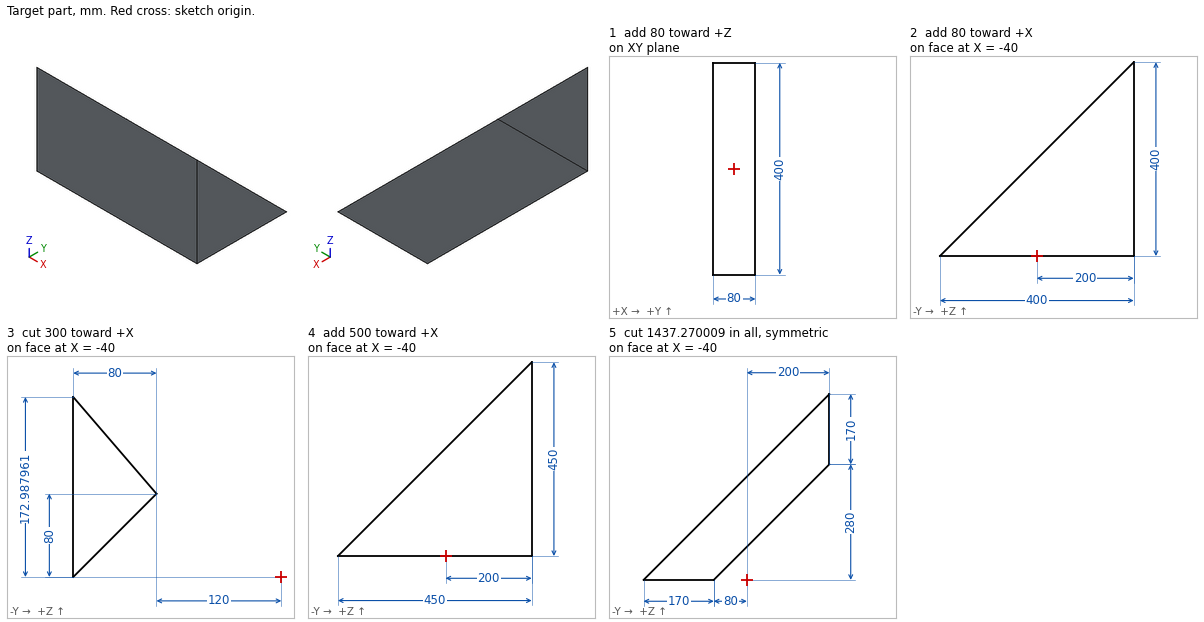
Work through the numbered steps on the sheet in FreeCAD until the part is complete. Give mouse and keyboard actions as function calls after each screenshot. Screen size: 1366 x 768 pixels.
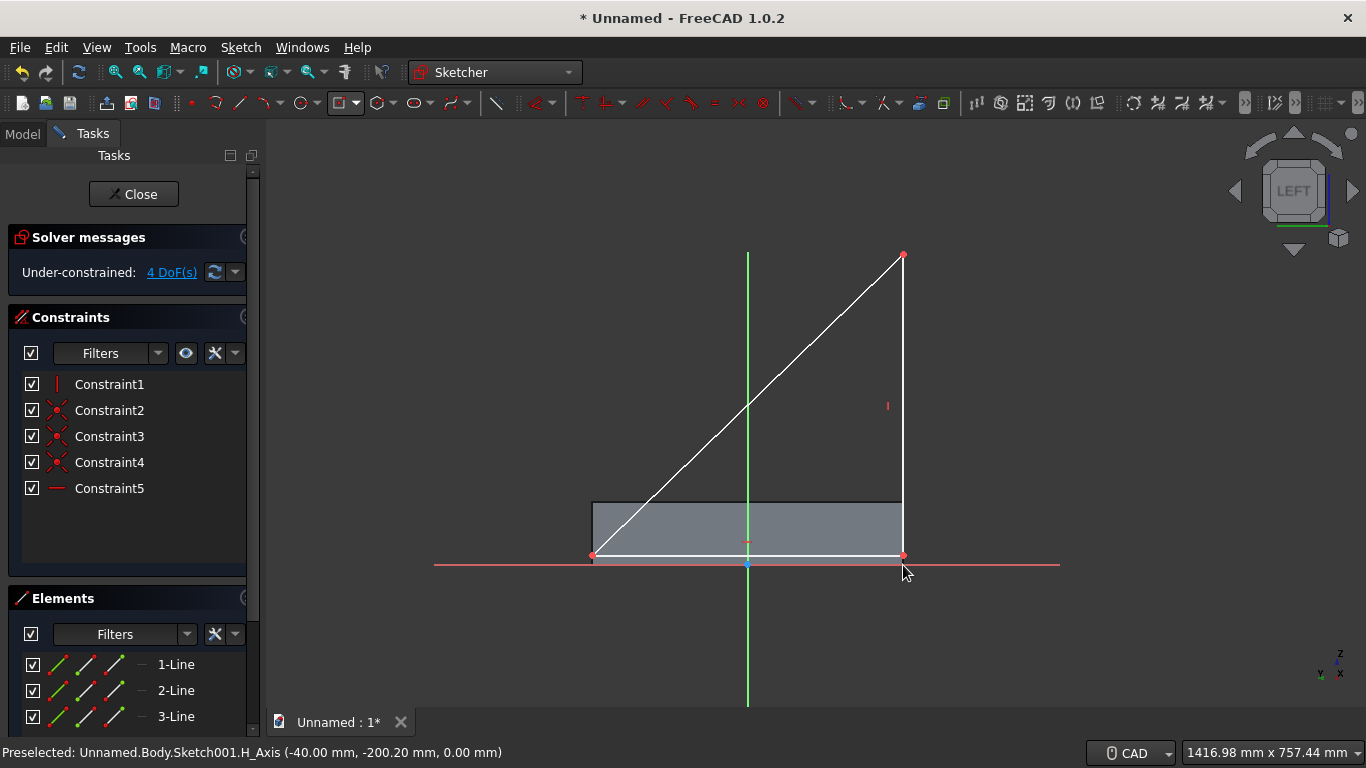
click(903, 556)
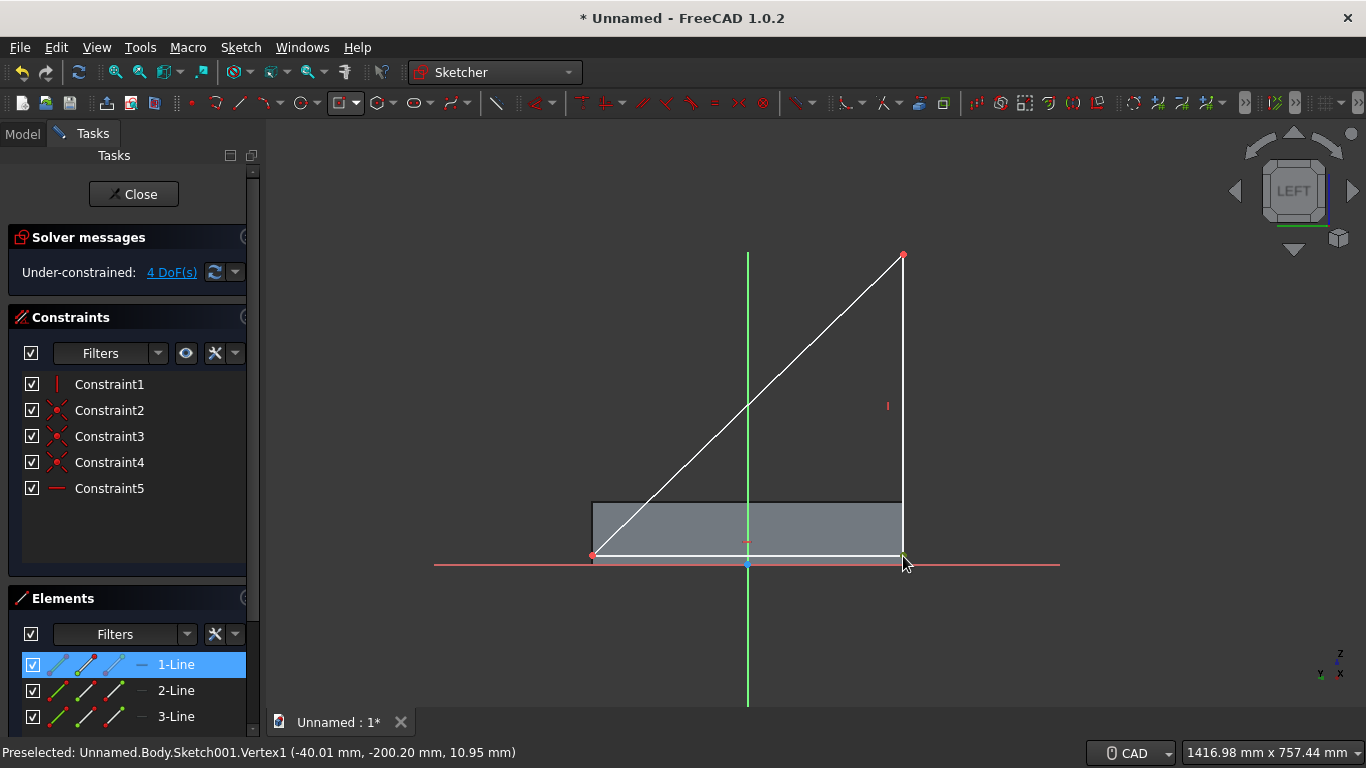
click(488, 564)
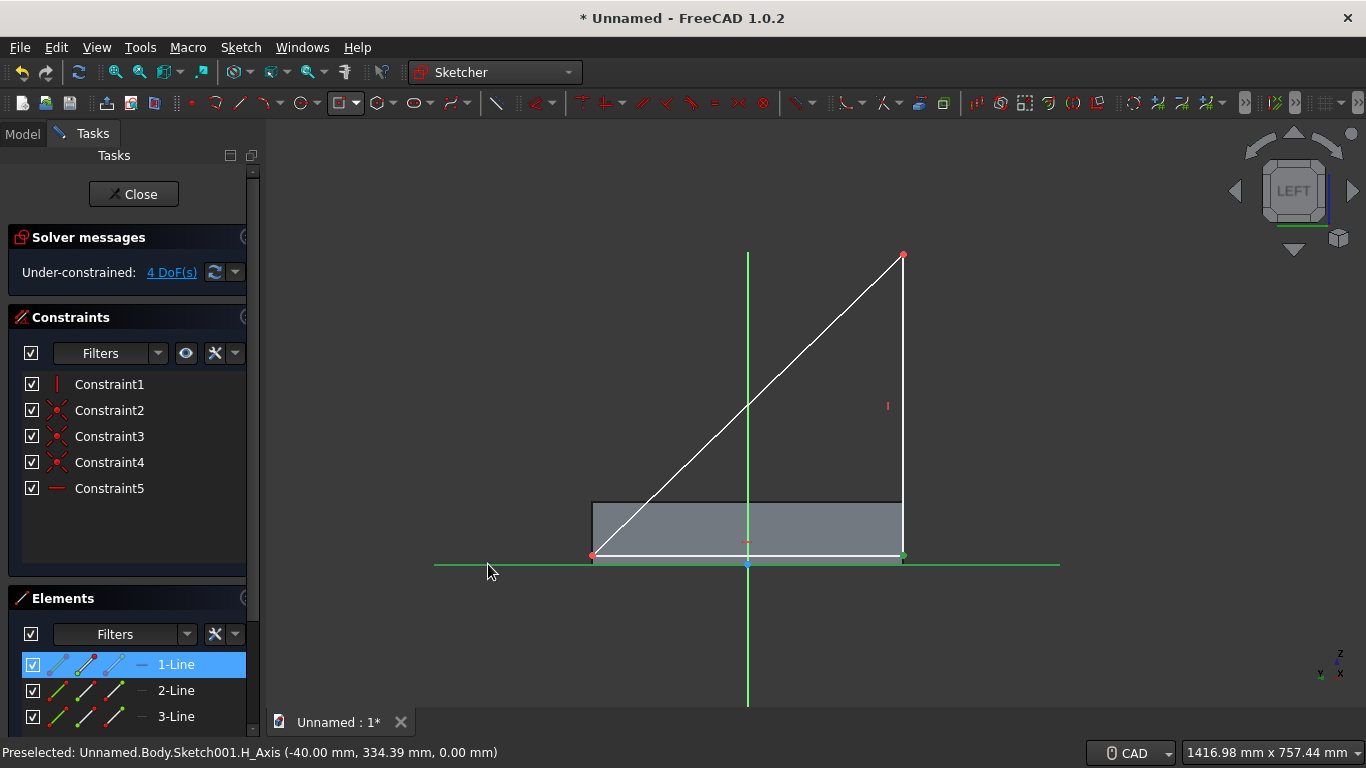
click(582, 104)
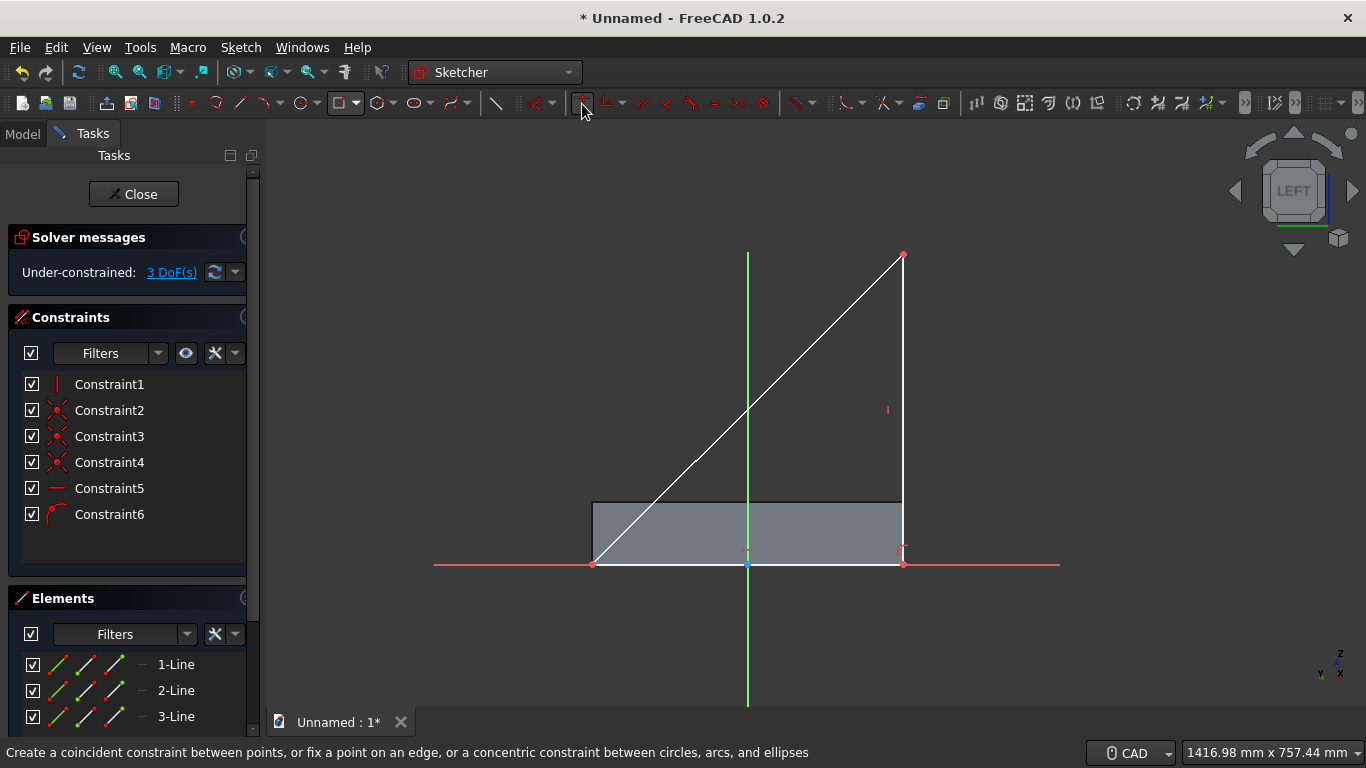
click(536, 104)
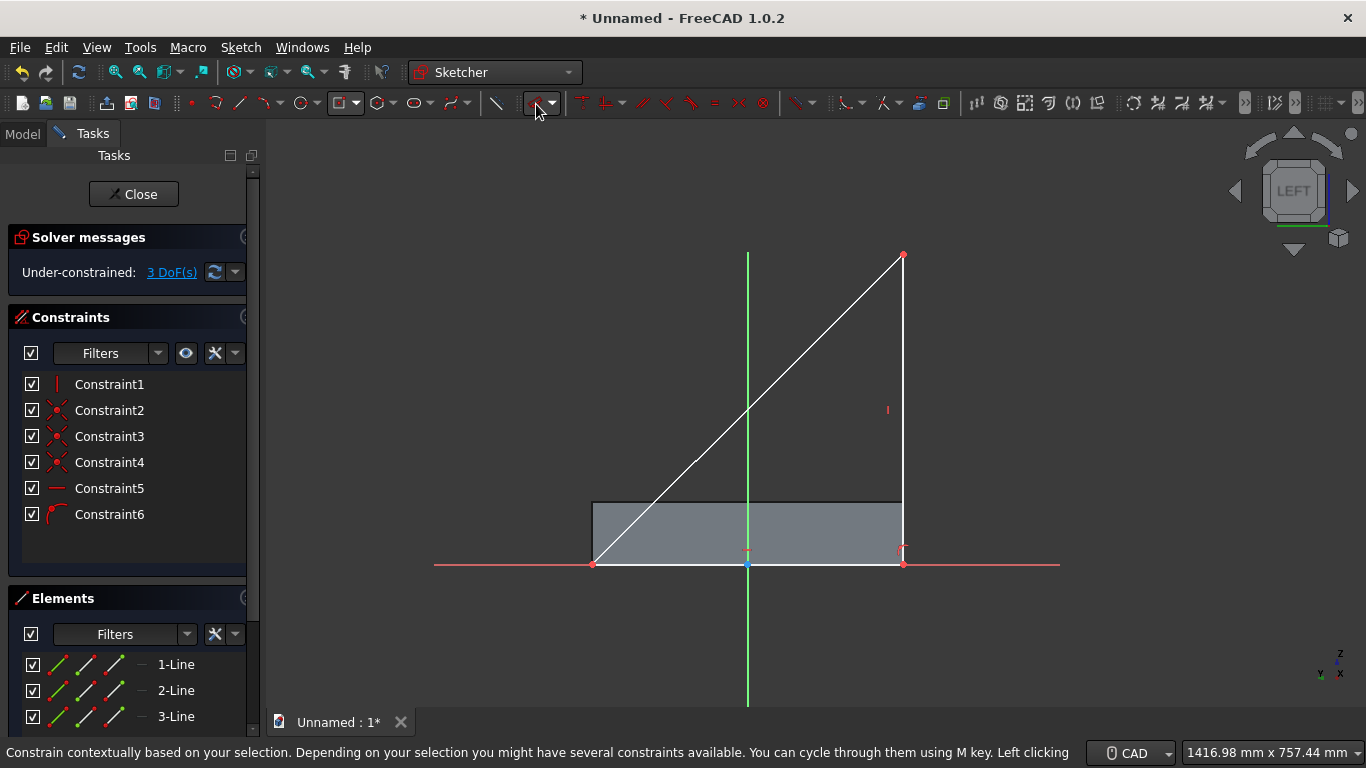
click(903, 472)
click(937, 410)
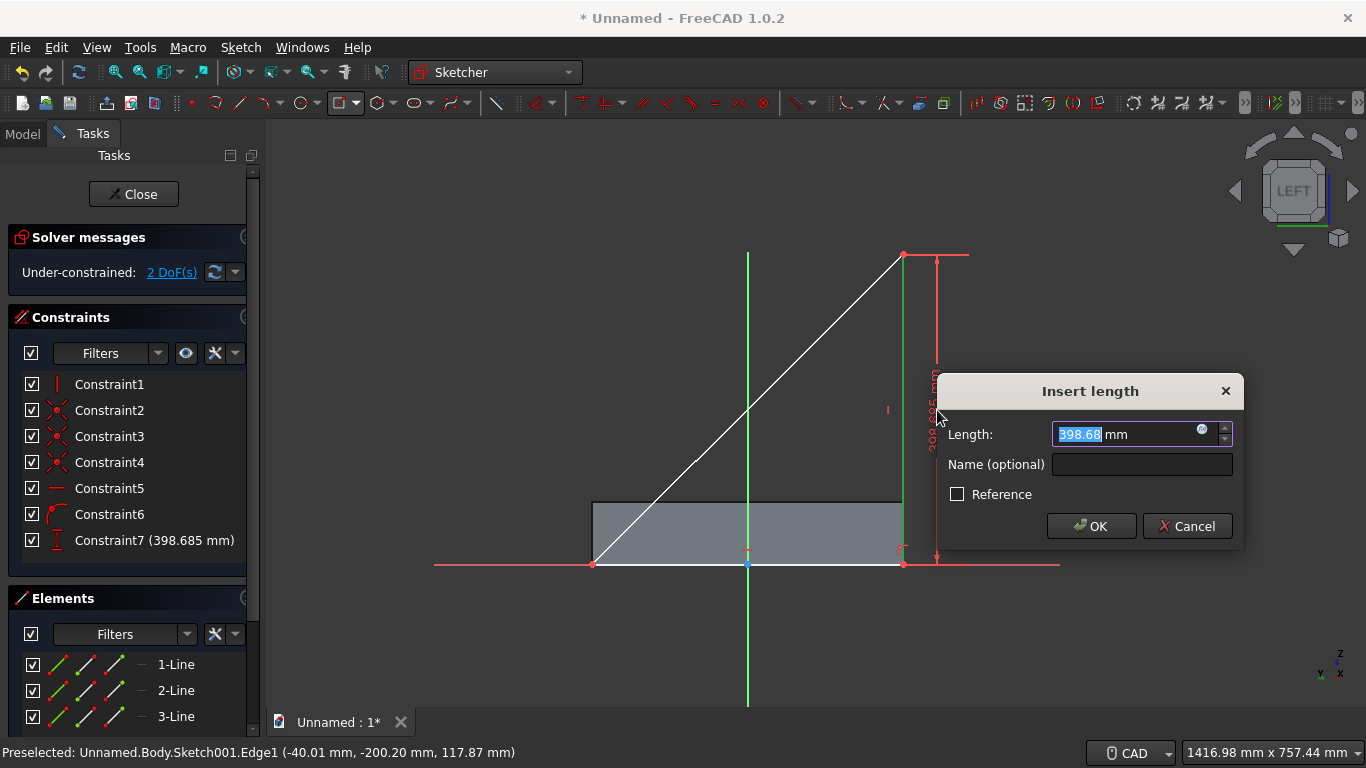
text(400)
key(Return)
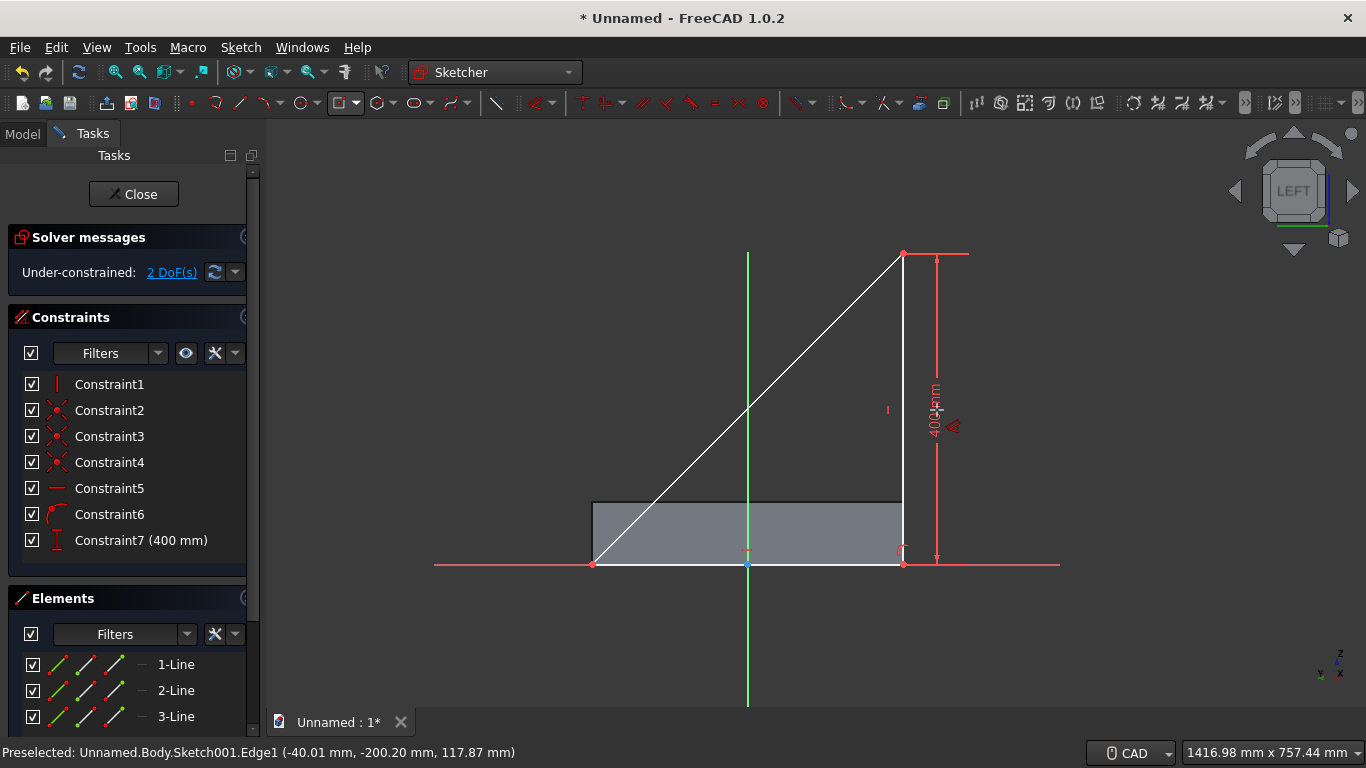
click(685, 564)
click(676, 598)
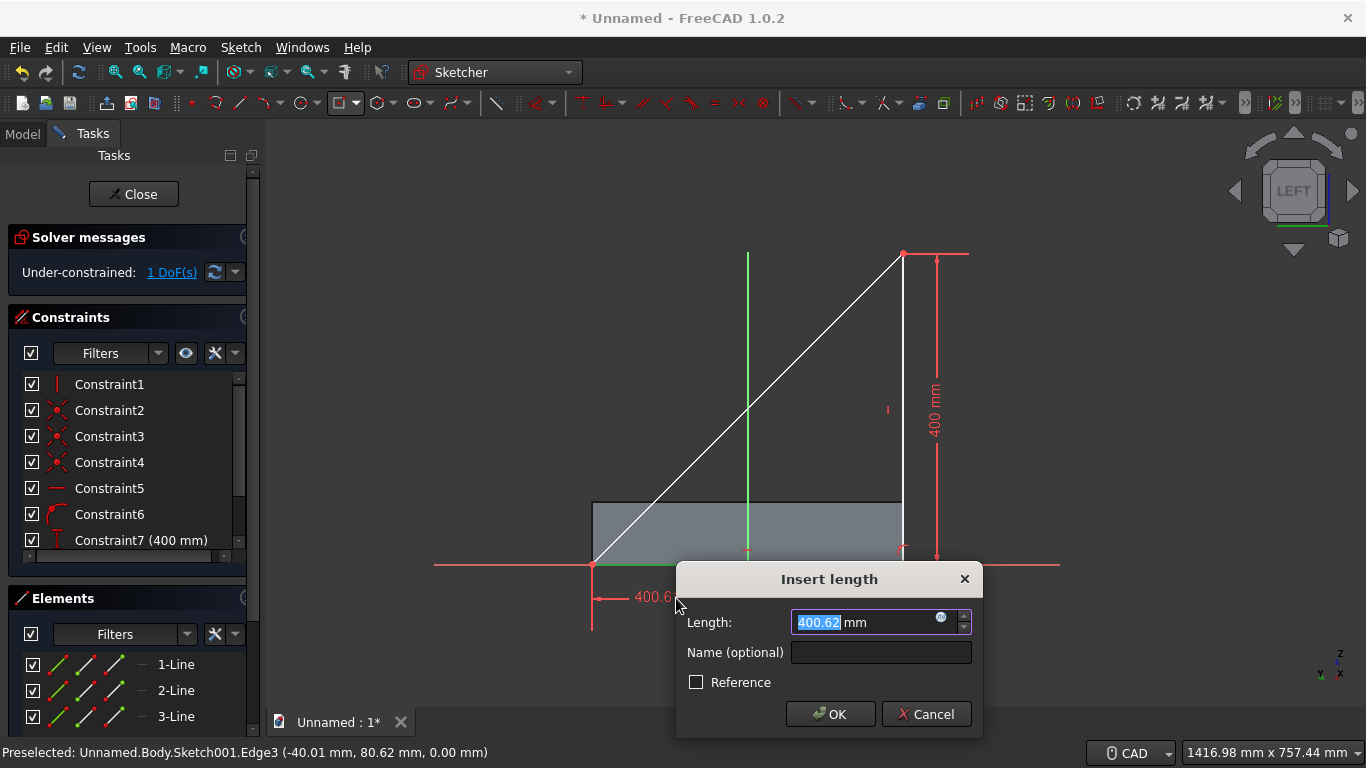
text(400)
key(Return)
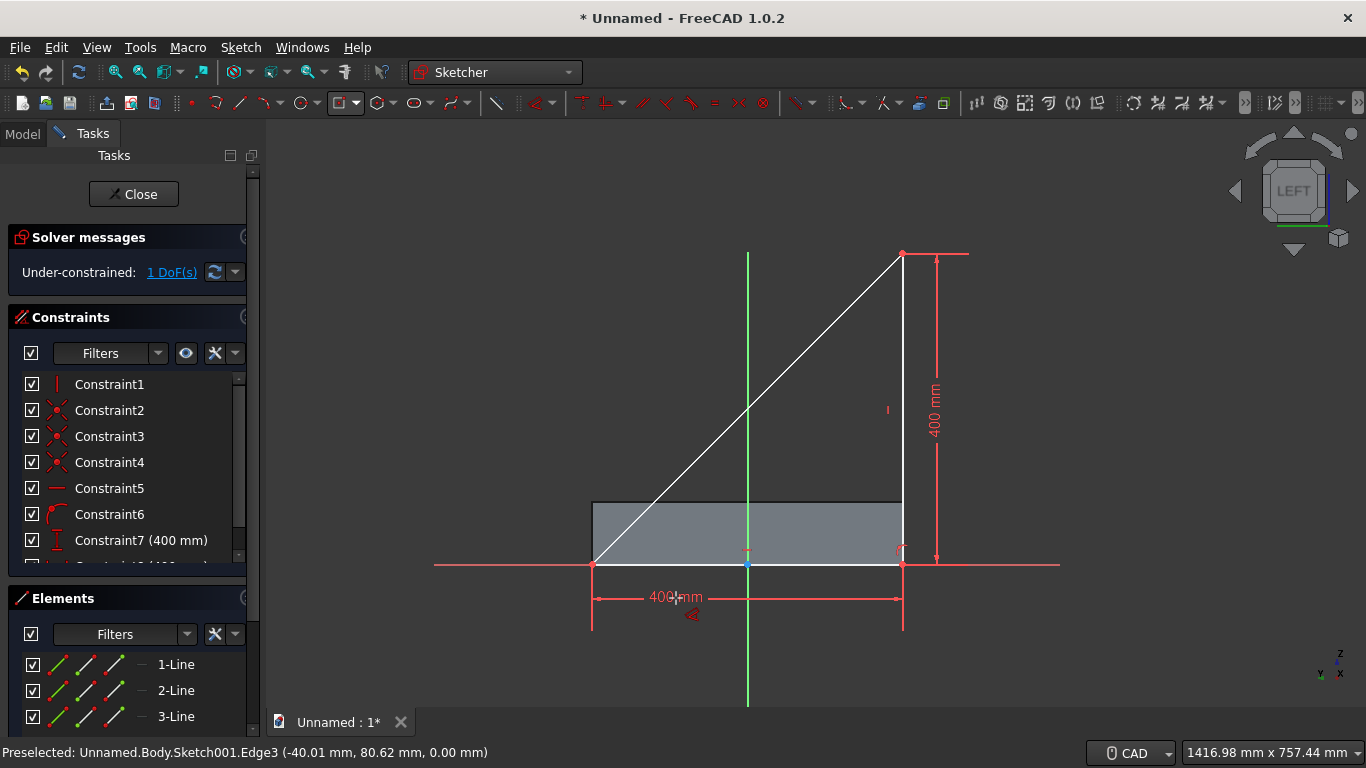
click(903, 564)
click(825, 598)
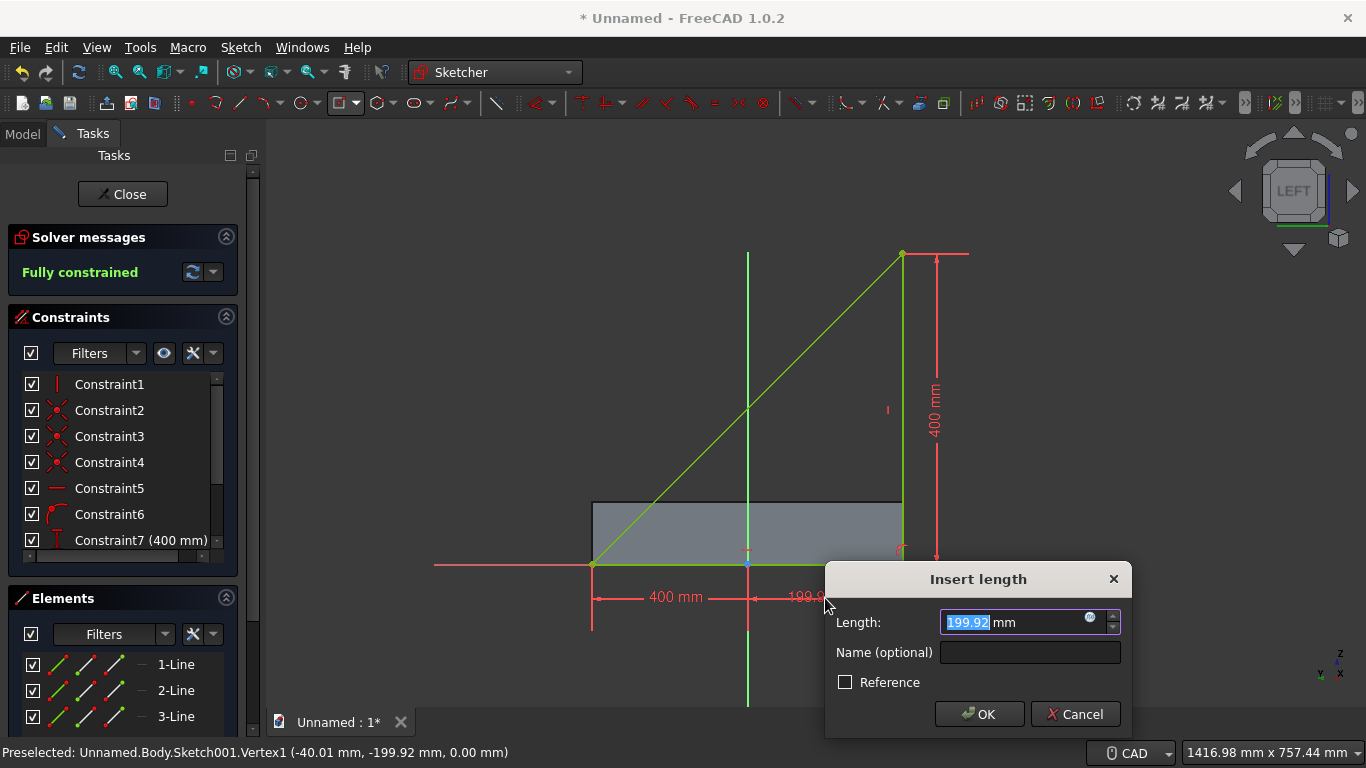
text(200)
key(Return)
key(Escape)